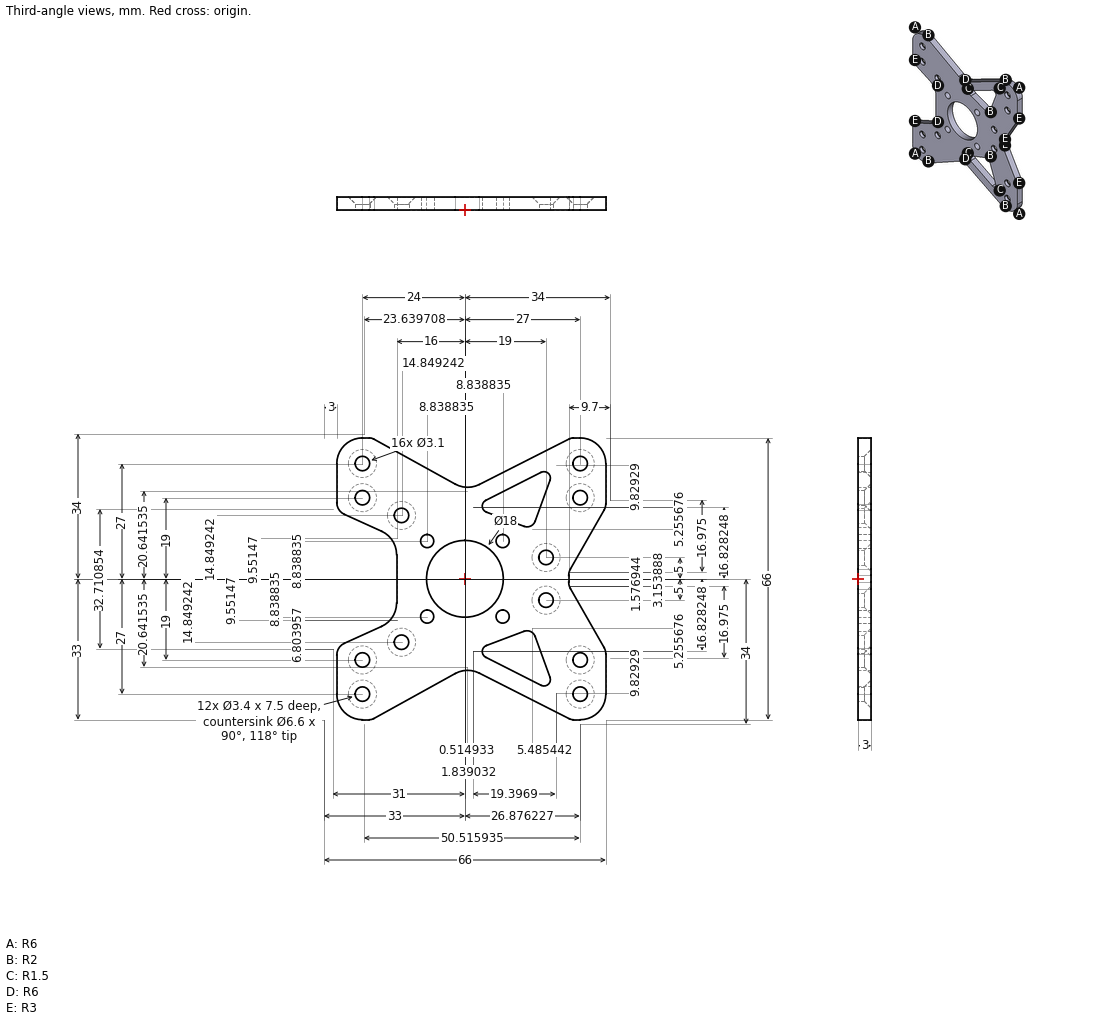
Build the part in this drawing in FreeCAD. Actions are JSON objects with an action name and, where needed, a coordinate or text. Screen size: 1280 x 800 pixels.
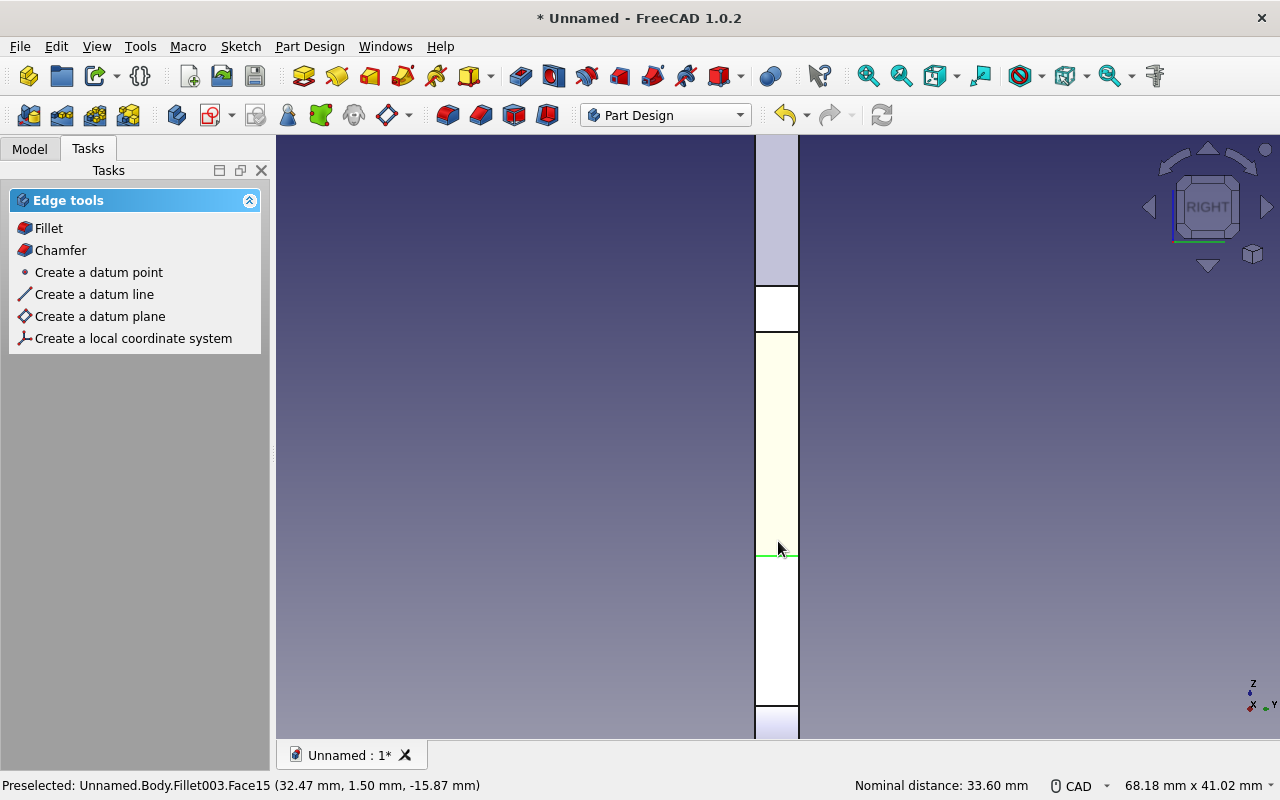
{"action": "left_click", "coordinate": [869, 76]}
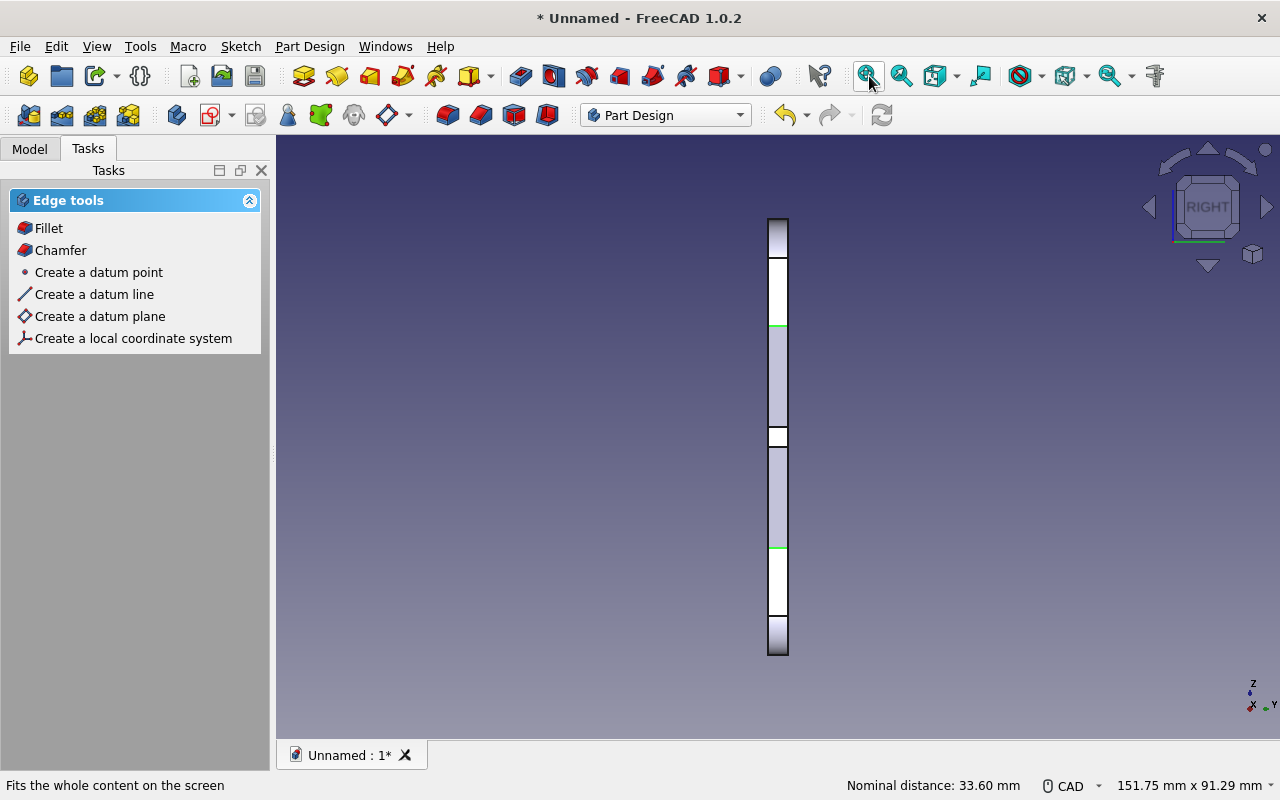
{"action": "key", "text": "5"}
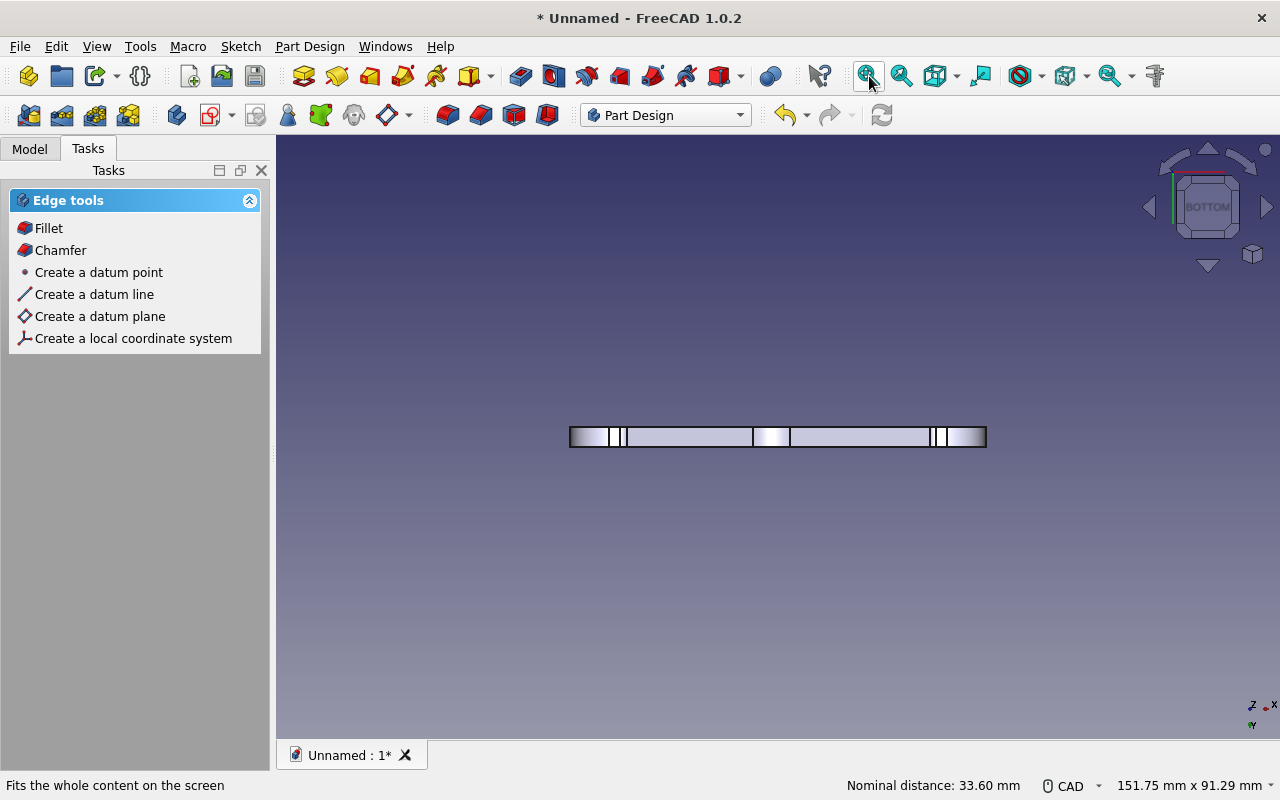
{"action": "left_click", "coordinate": [869, 76]}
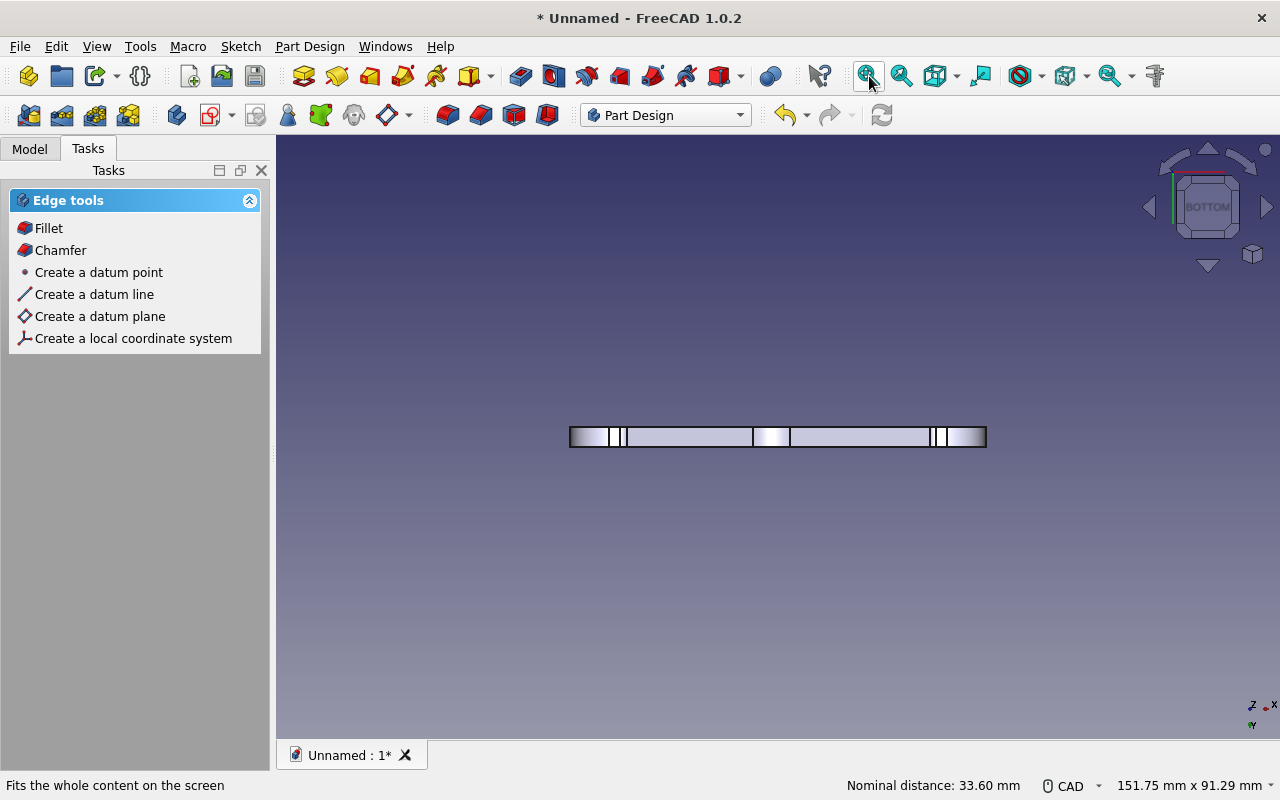
{"action": "scroll", "coordinate": [570, 436], "scroll_direction": "up", "scroll_amount": 4}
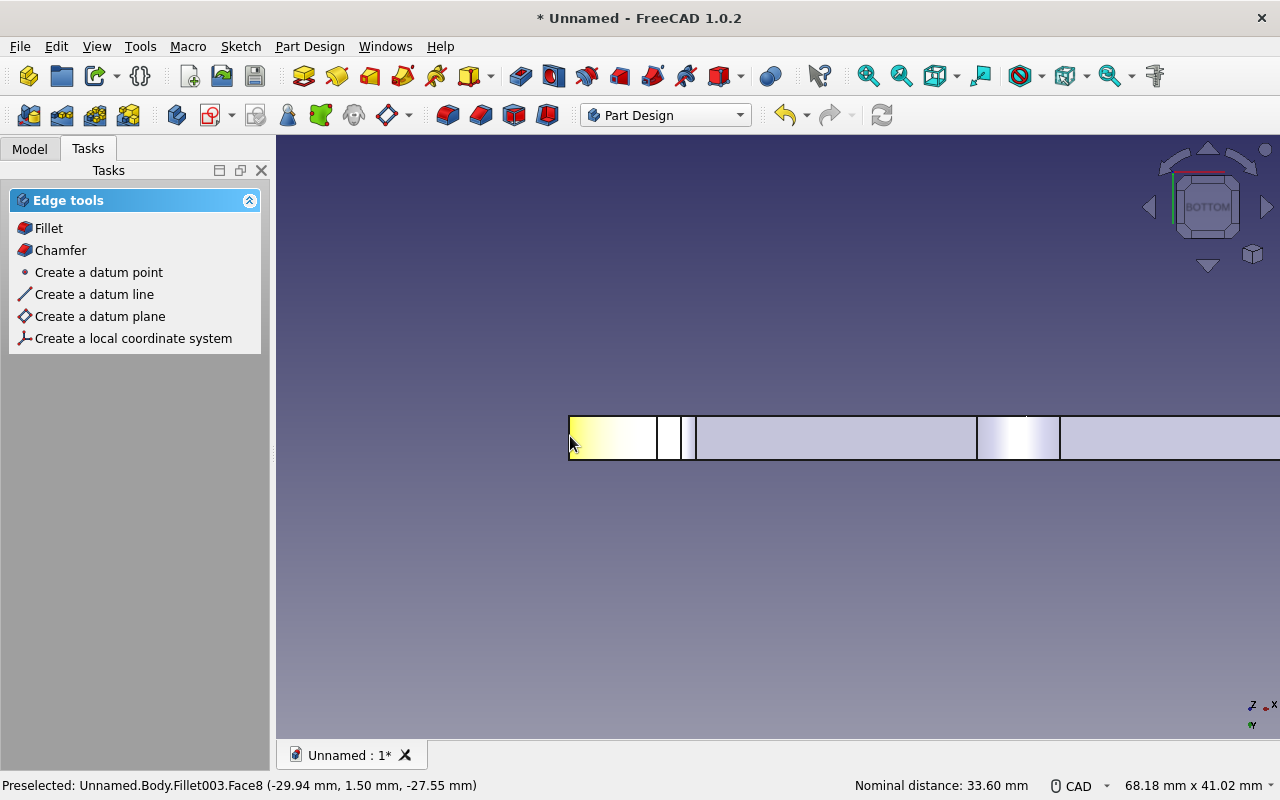
{"action": "left_click", "coordinate": [869, 76]}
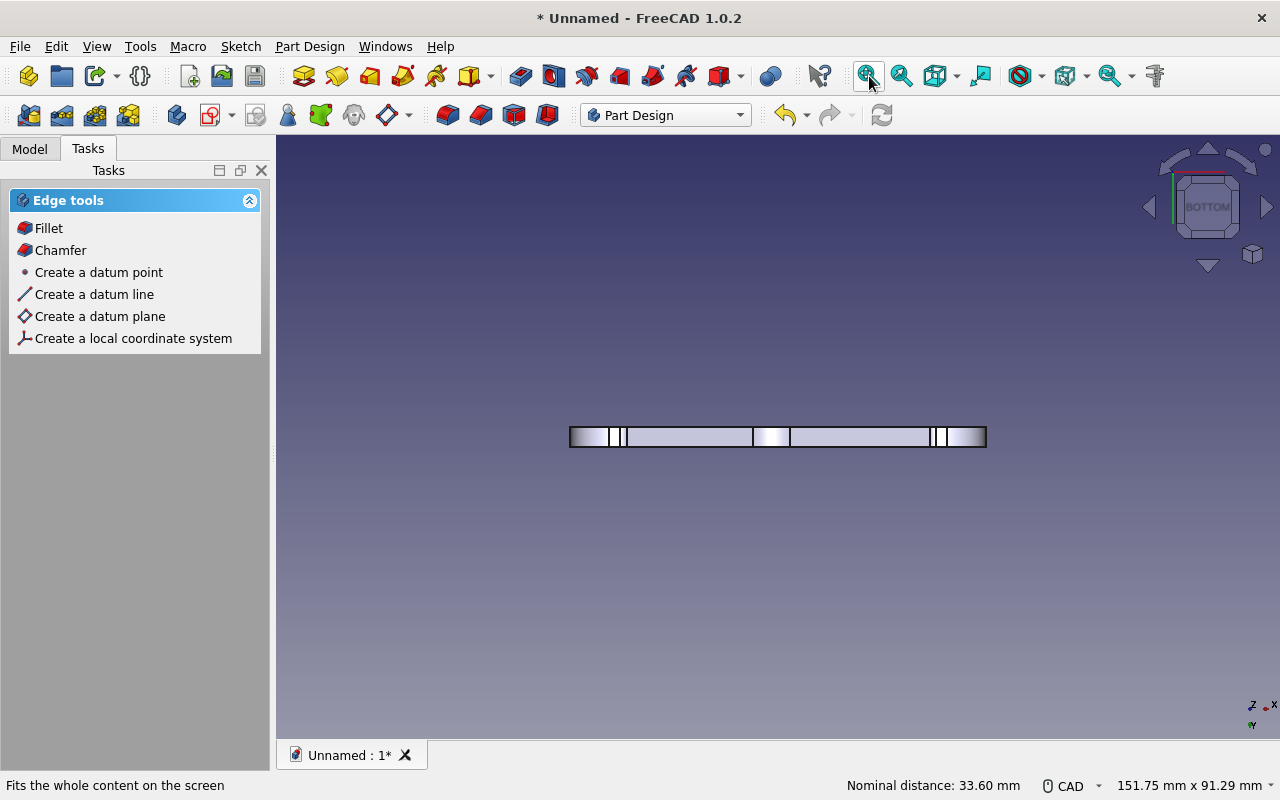
{"action": "key", "text": "4"}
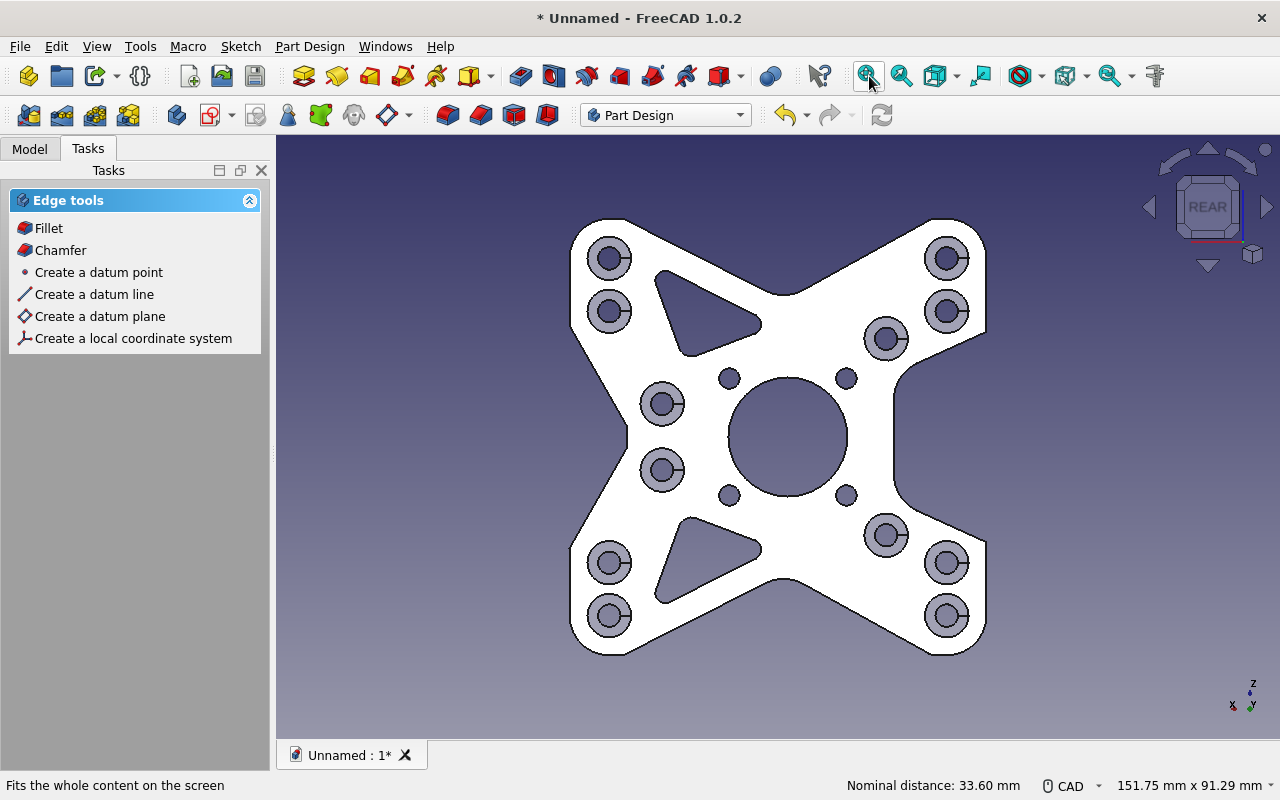
{"action": "scroll", "coordinate": [986, 541], "scroll_direction": "up", "scroll_amount": 4}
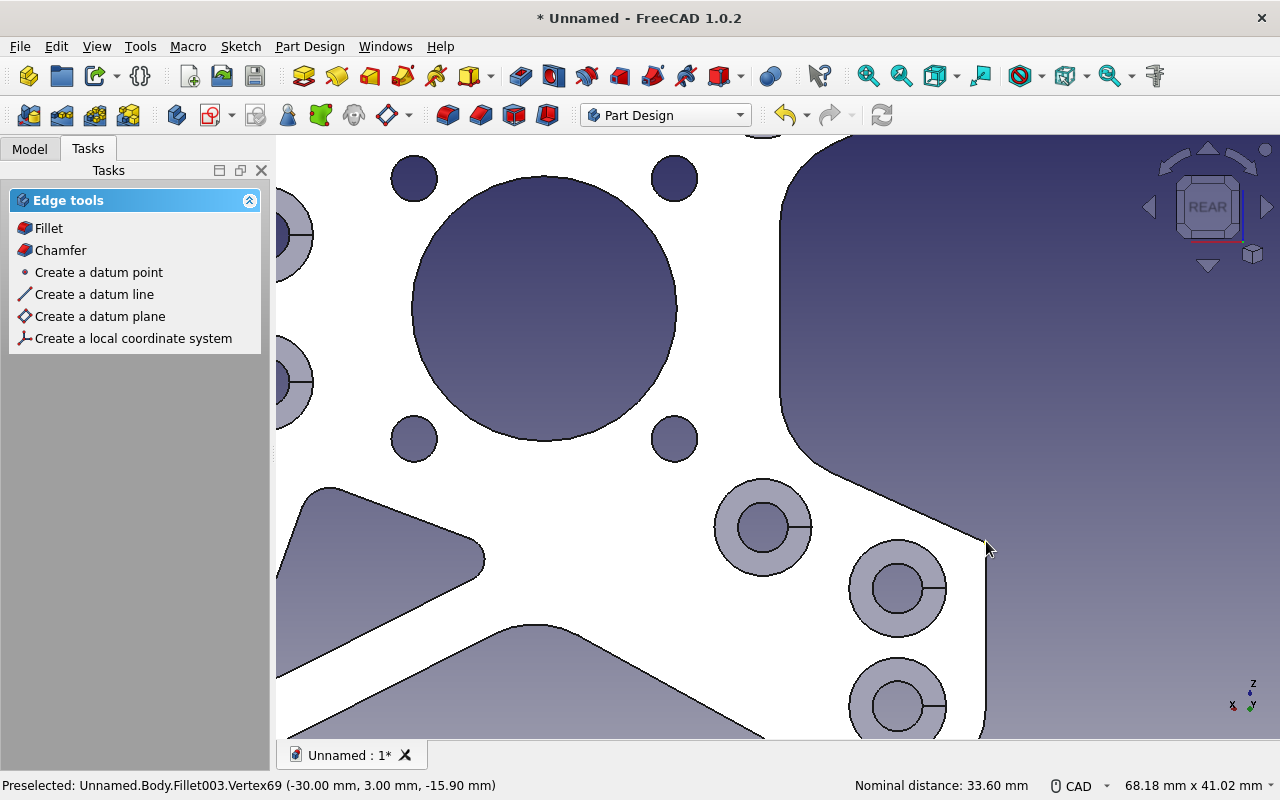
{"action": "key", "text": "v f"}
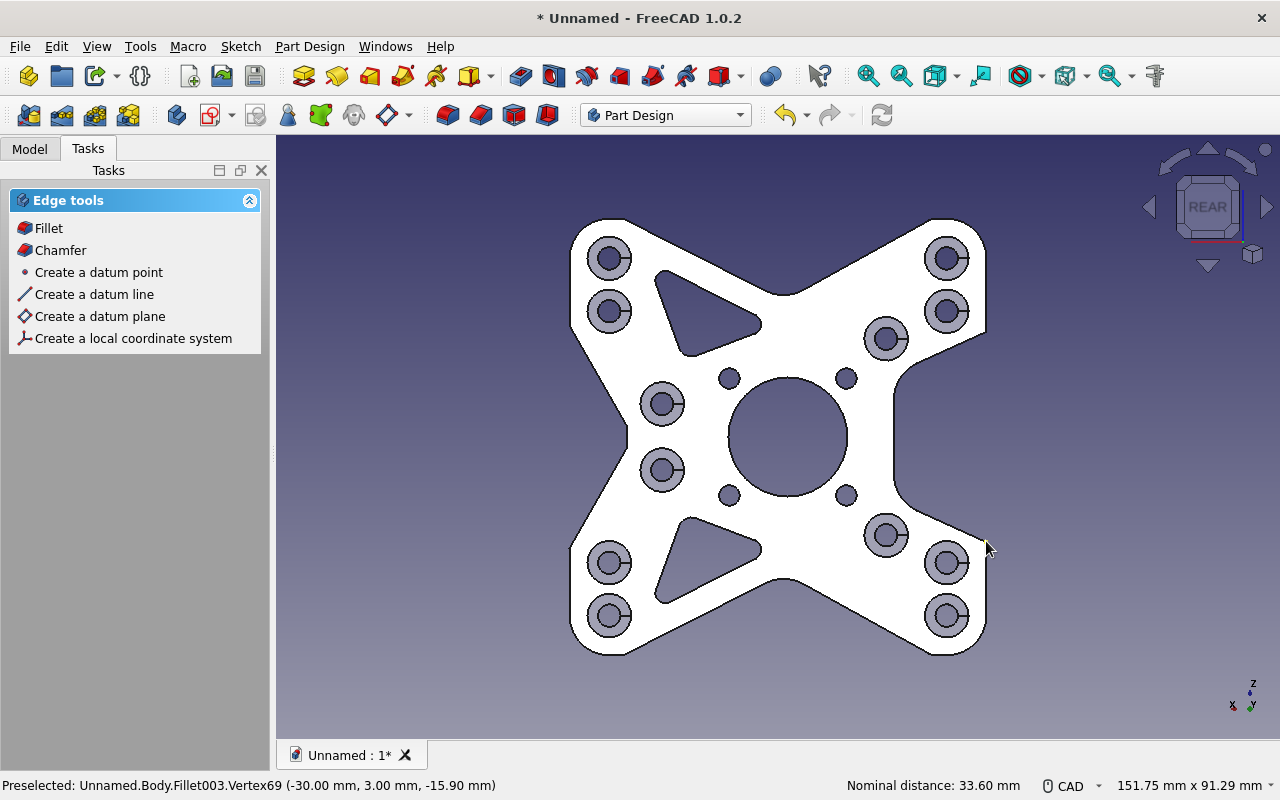
{"action": "key", "text": "6"}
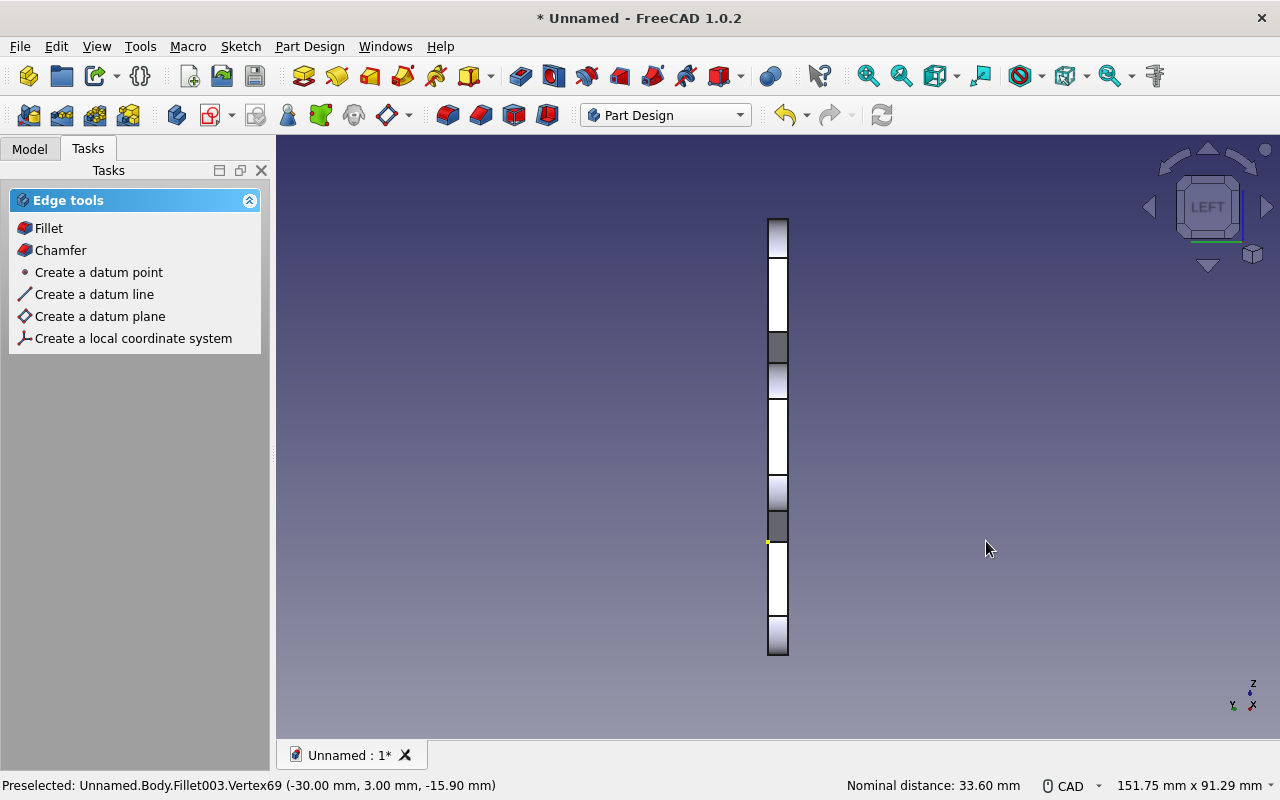
{"action": "left_click", "coordinate": [778, 541], "text": "ctrl"}